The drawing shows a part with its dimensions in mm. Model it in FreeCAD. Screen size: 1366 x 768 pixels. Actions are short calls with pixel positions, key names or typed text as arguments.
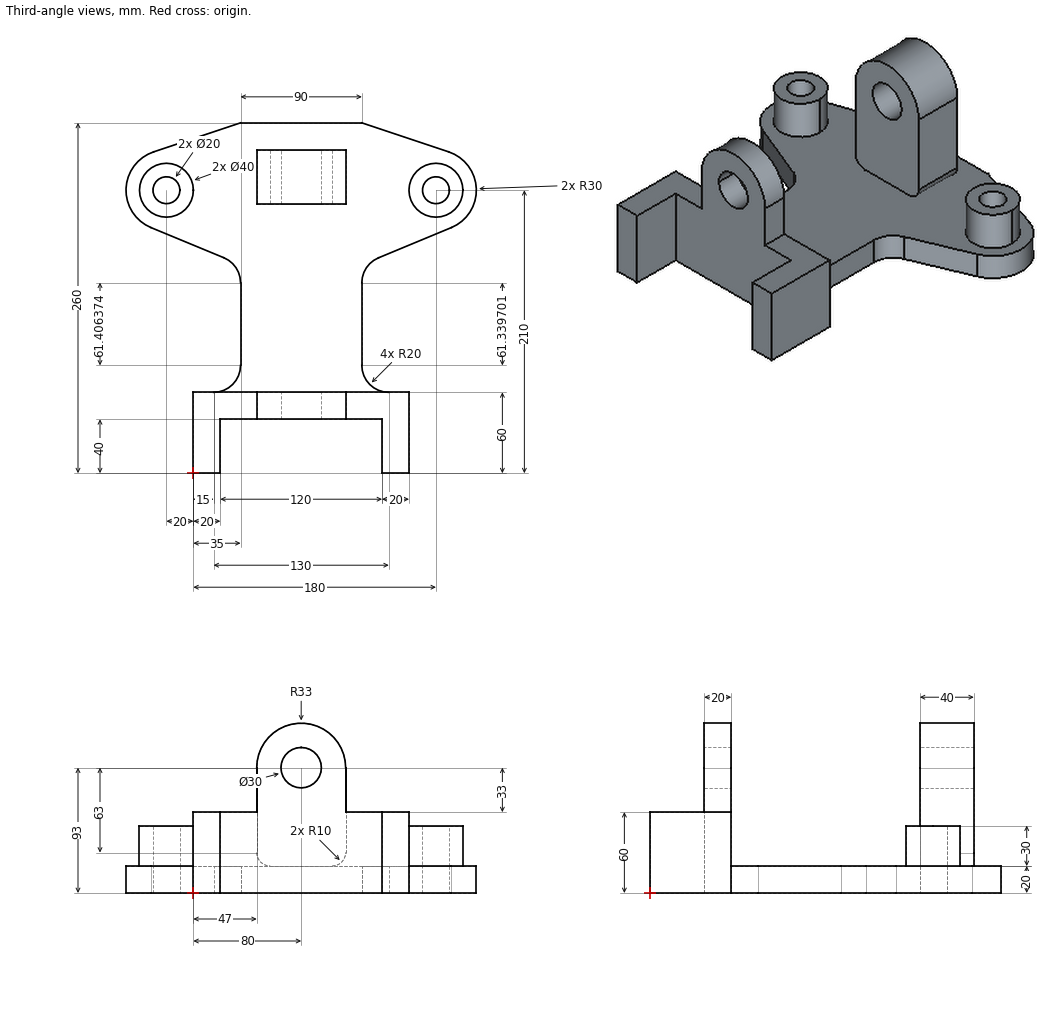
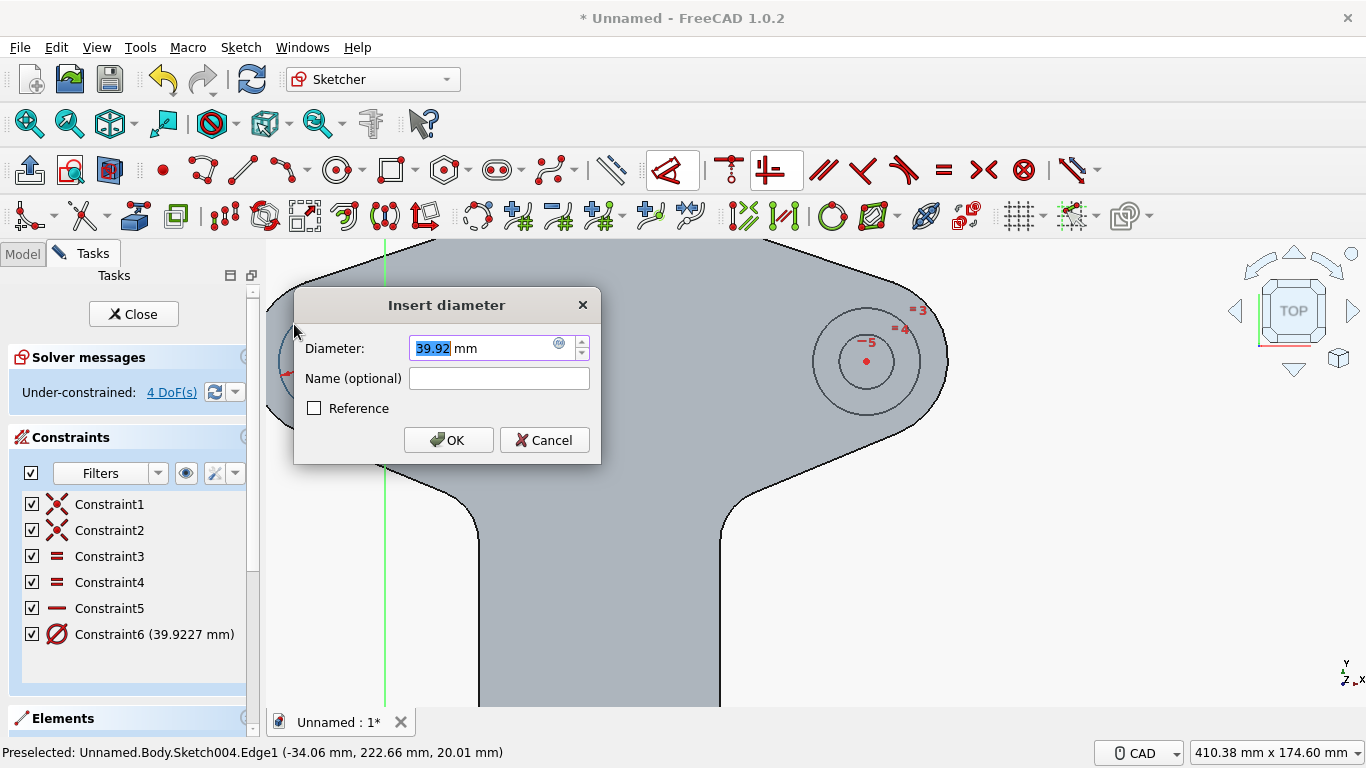
text(40)
key(Return)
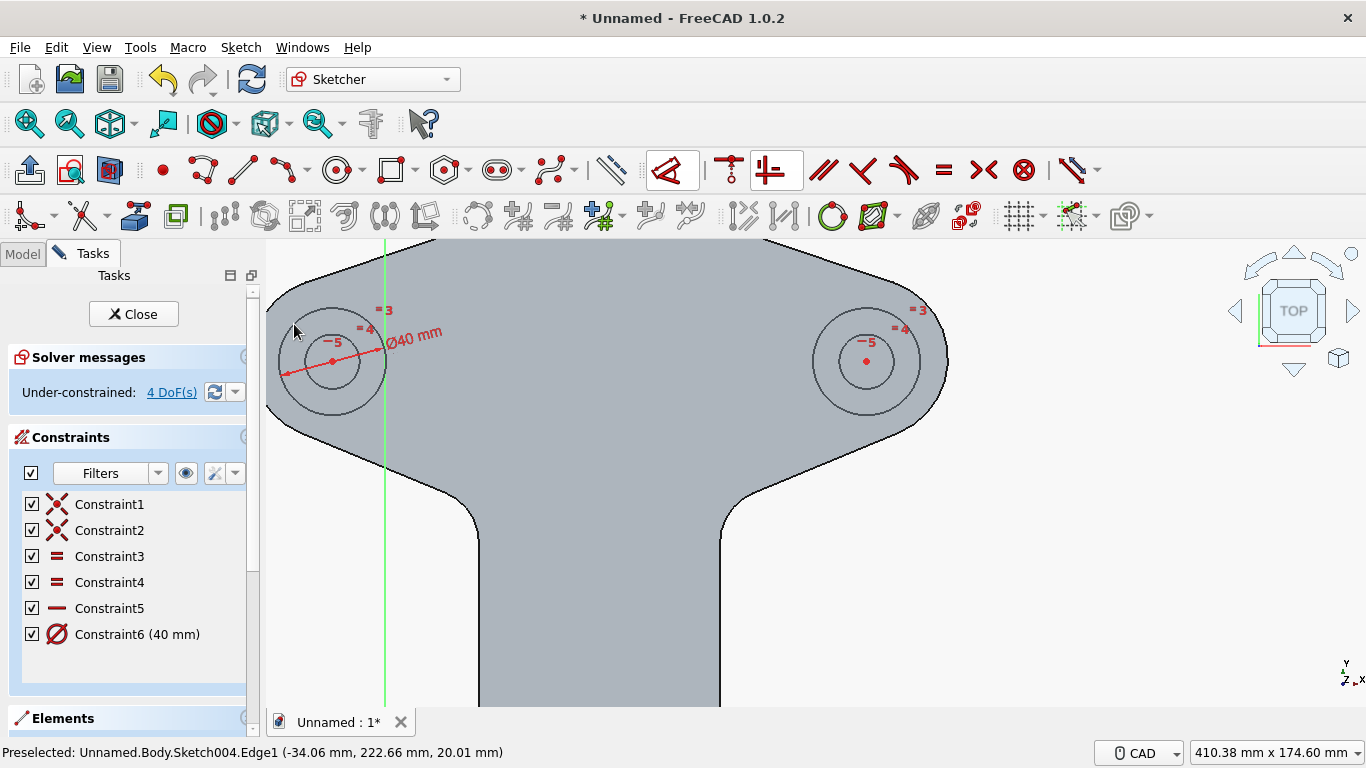
click(352, 342)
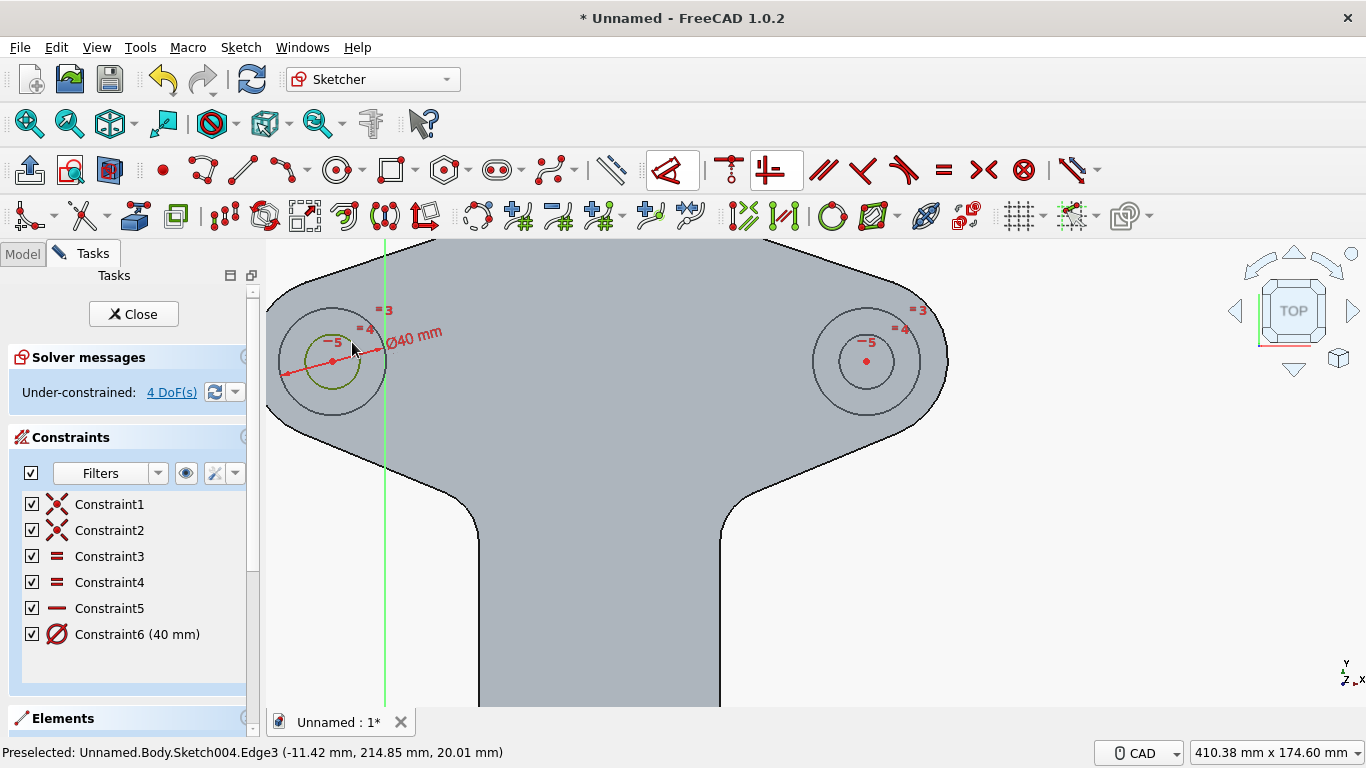
click(694, 170)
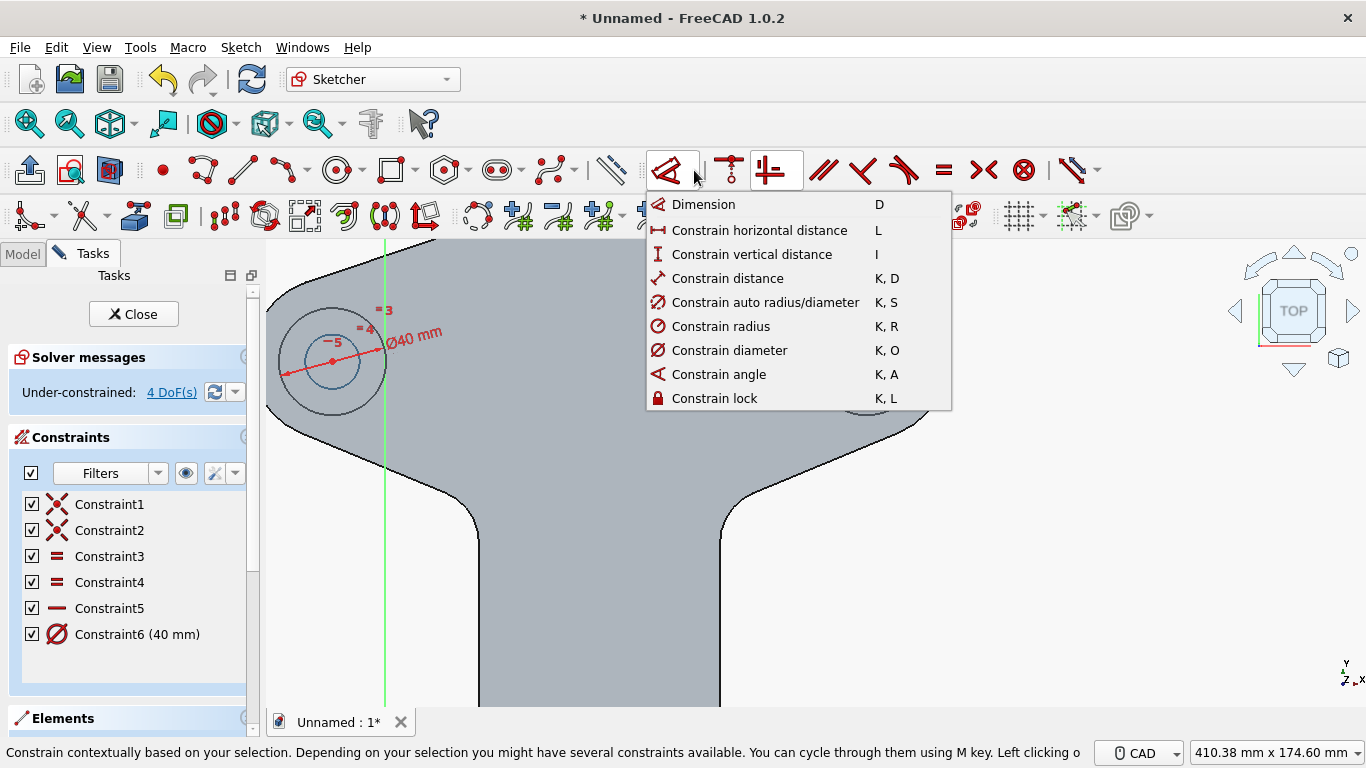
click(799, 350)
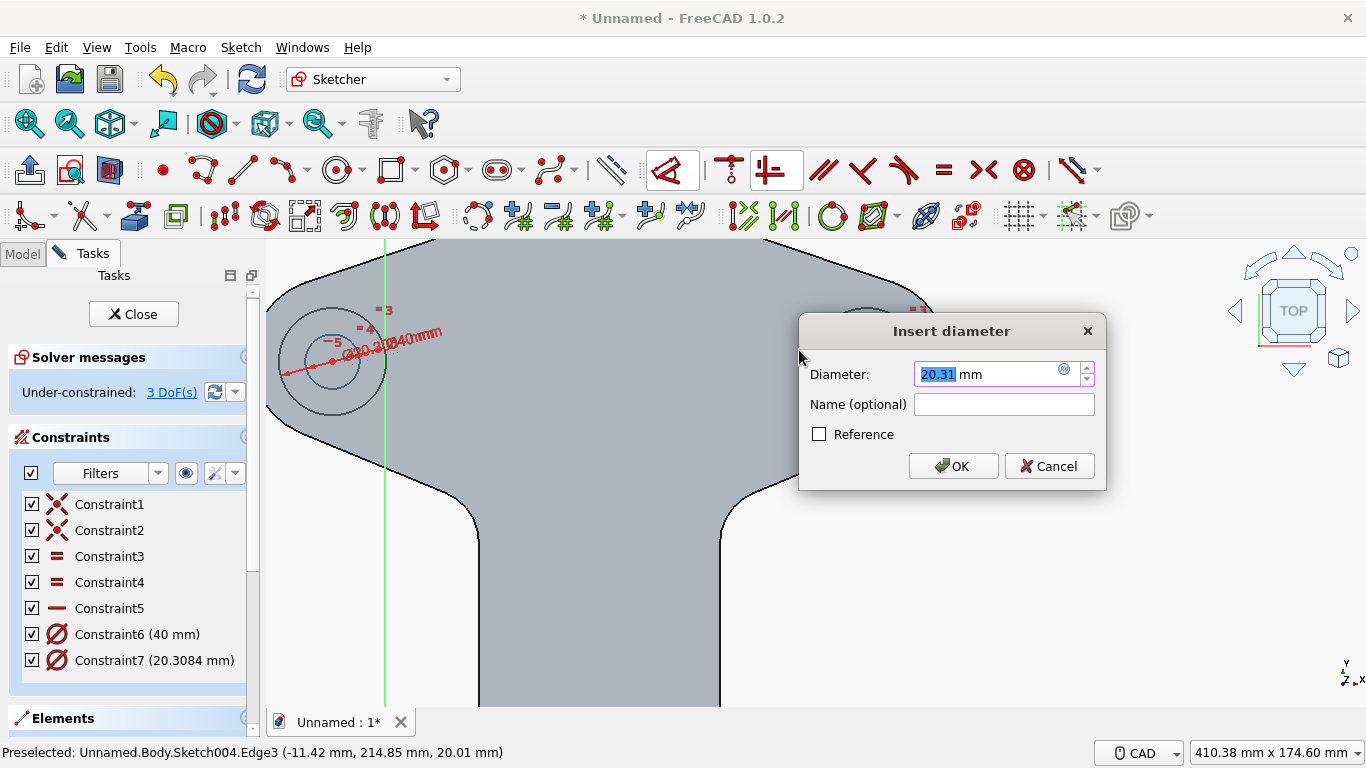
text(20)
key(Return)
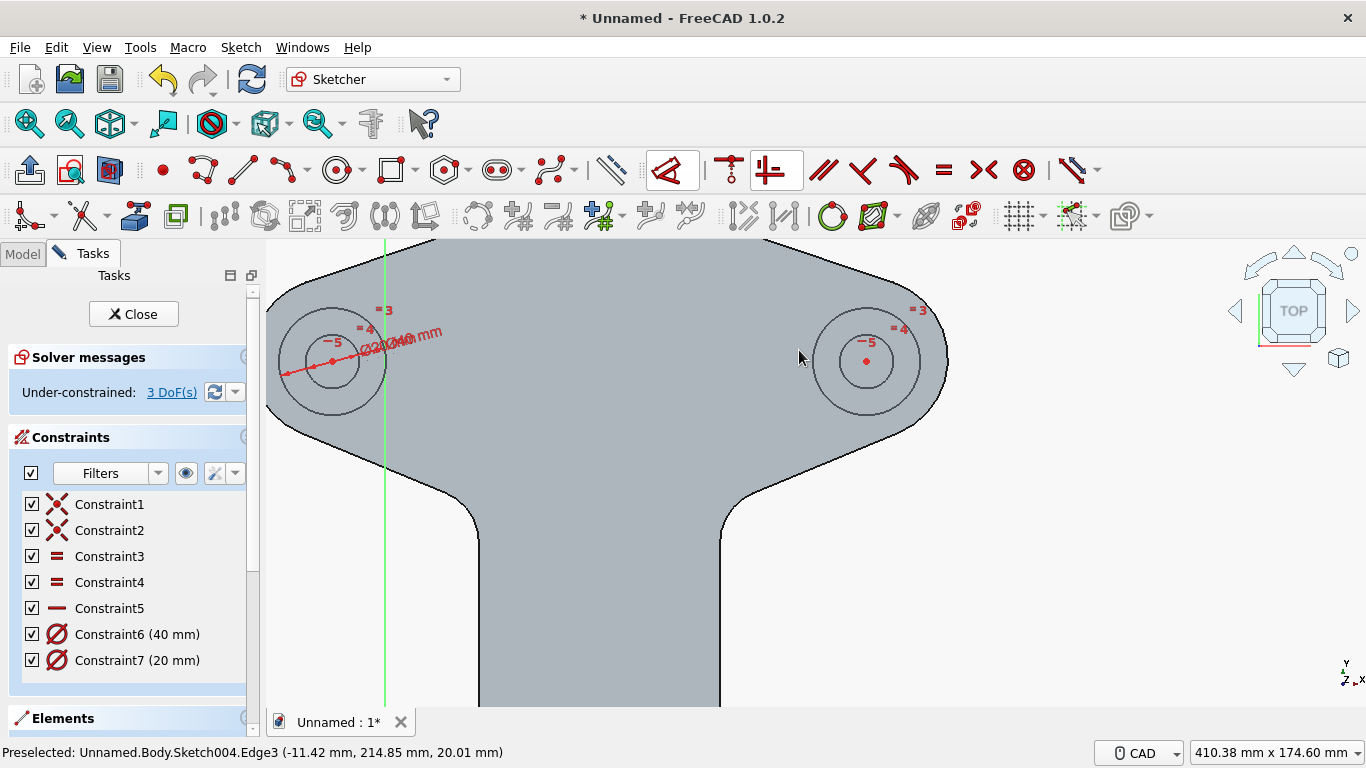
click(332, 362)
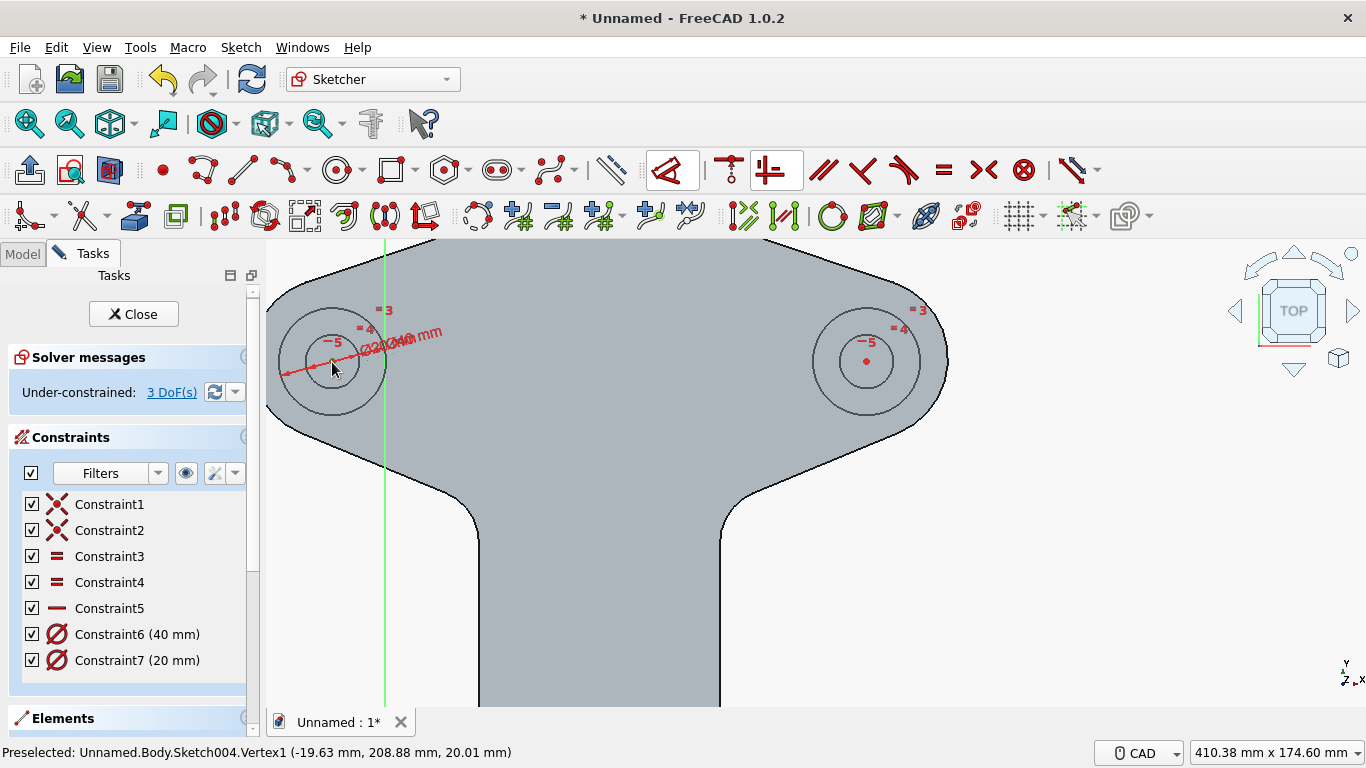
click(694, 170)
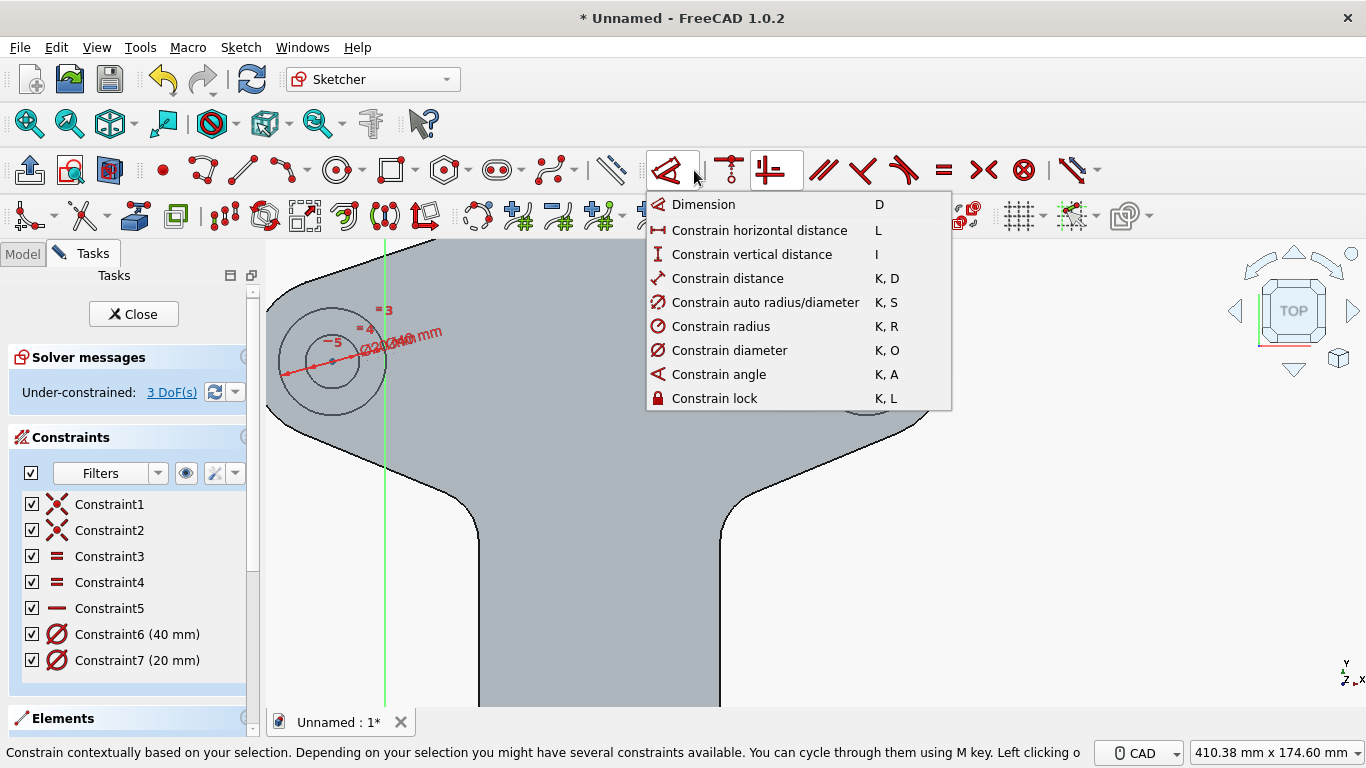
click(799, 230)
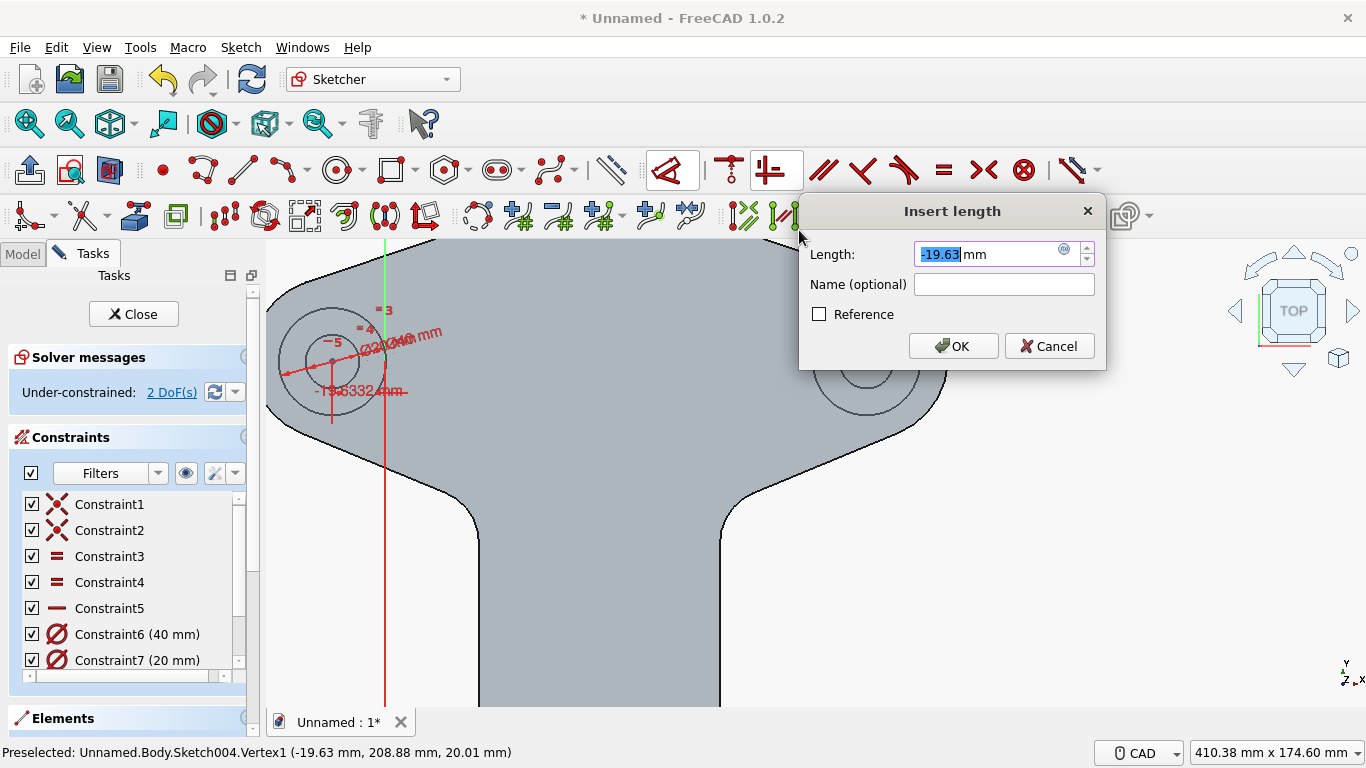
text(-20)
key(Return)